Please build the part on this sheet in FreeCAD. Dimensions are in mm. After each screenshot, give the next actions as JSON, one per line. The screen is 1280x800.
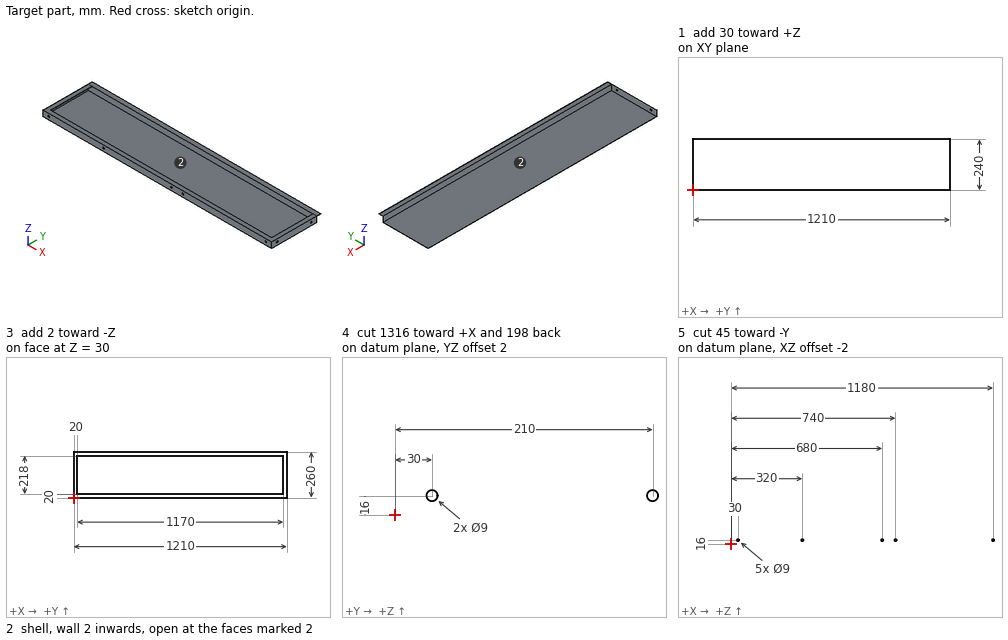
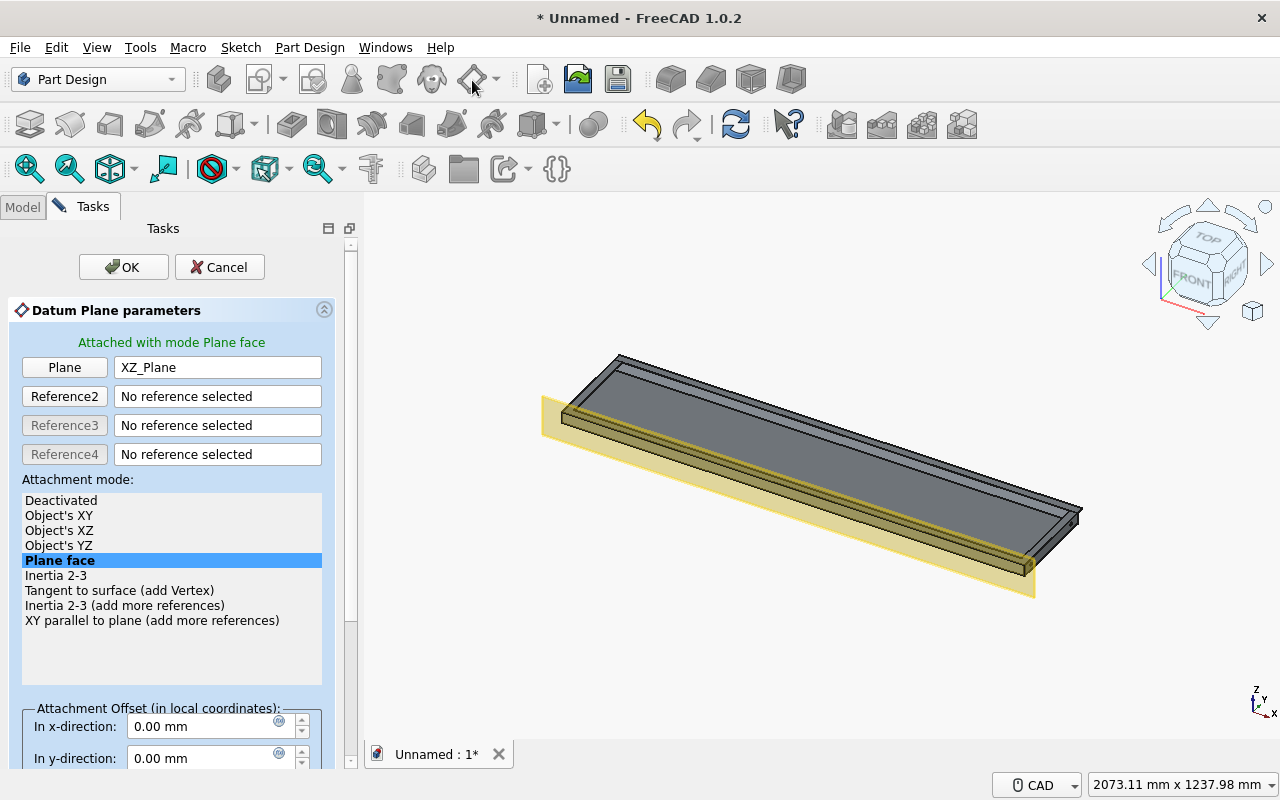
{"action": "scroll", "coordinate": [351, 503], "scroll_direction": "down", "scroll_amount": 2}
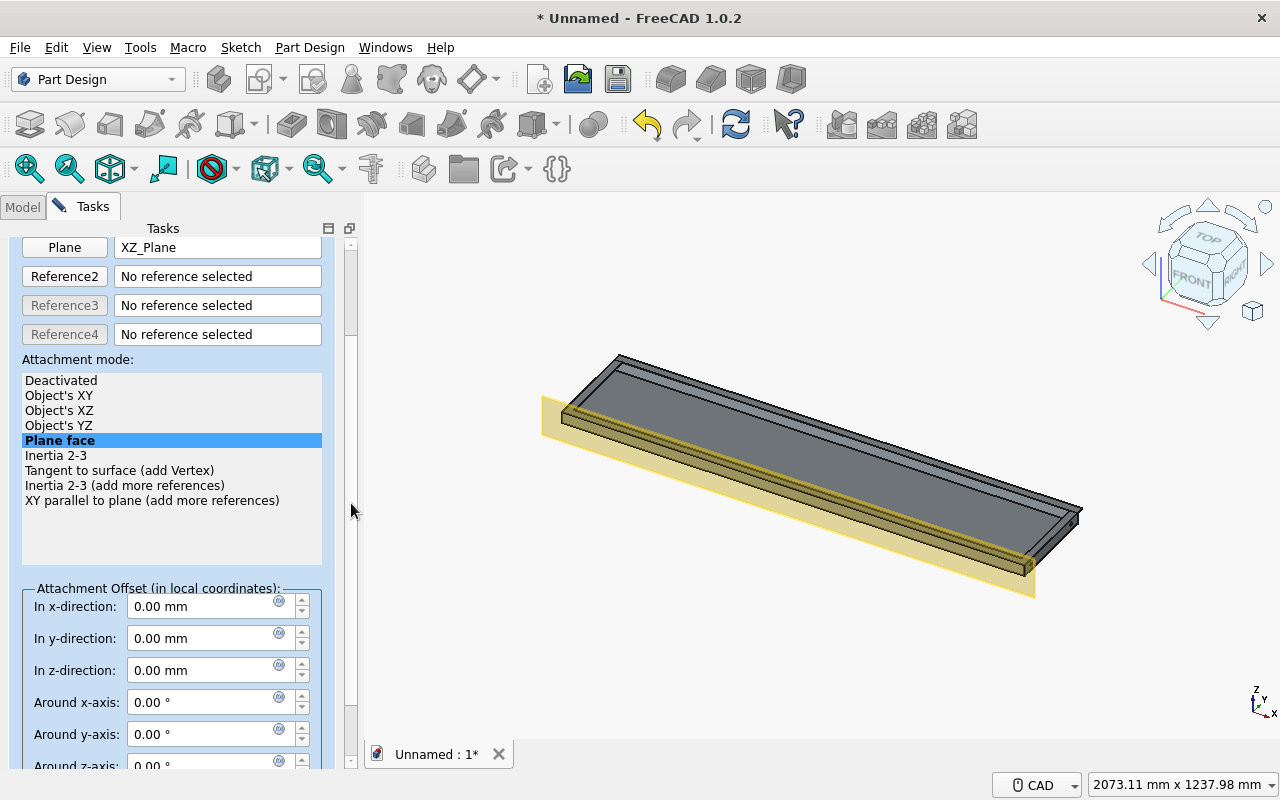
{"action": "triple_click", "coordinate": [210, 670]}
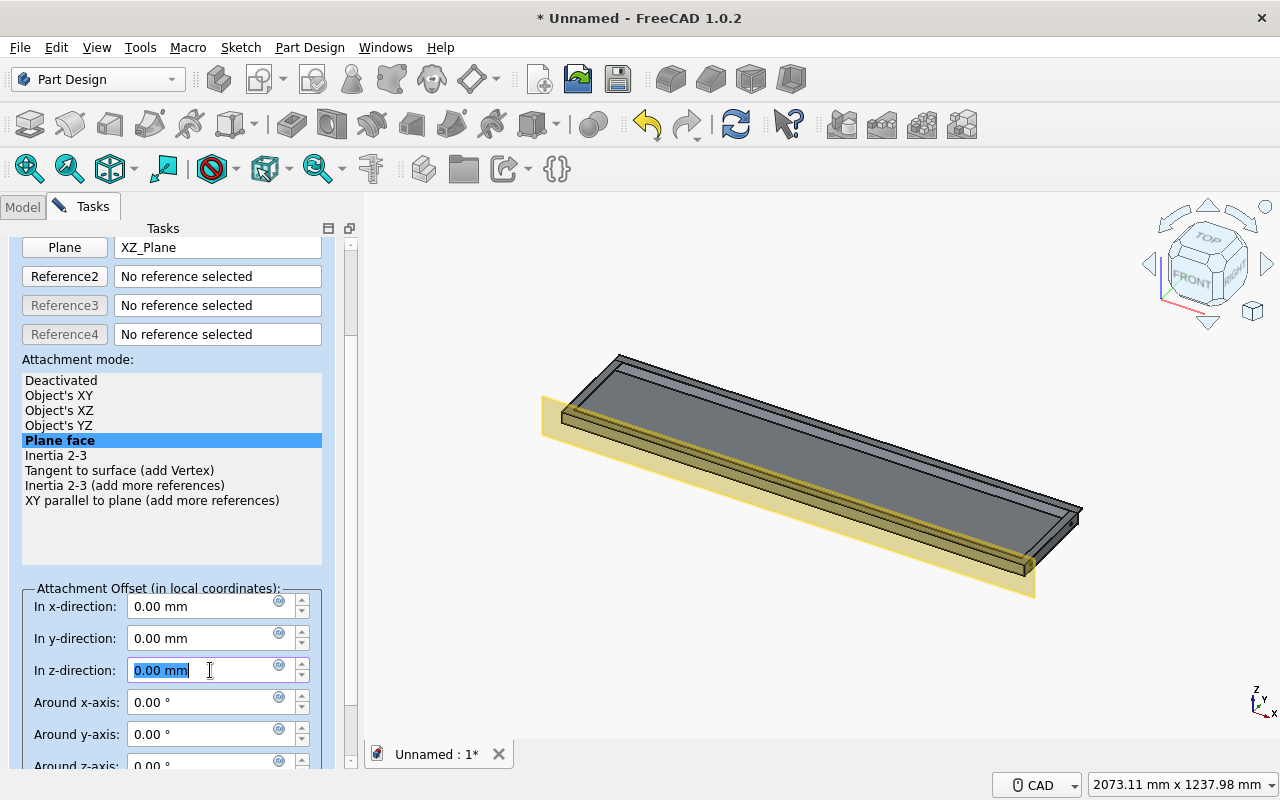
{"action": "type", "text": "-2"}
{"action": "key", "text": "Tab"}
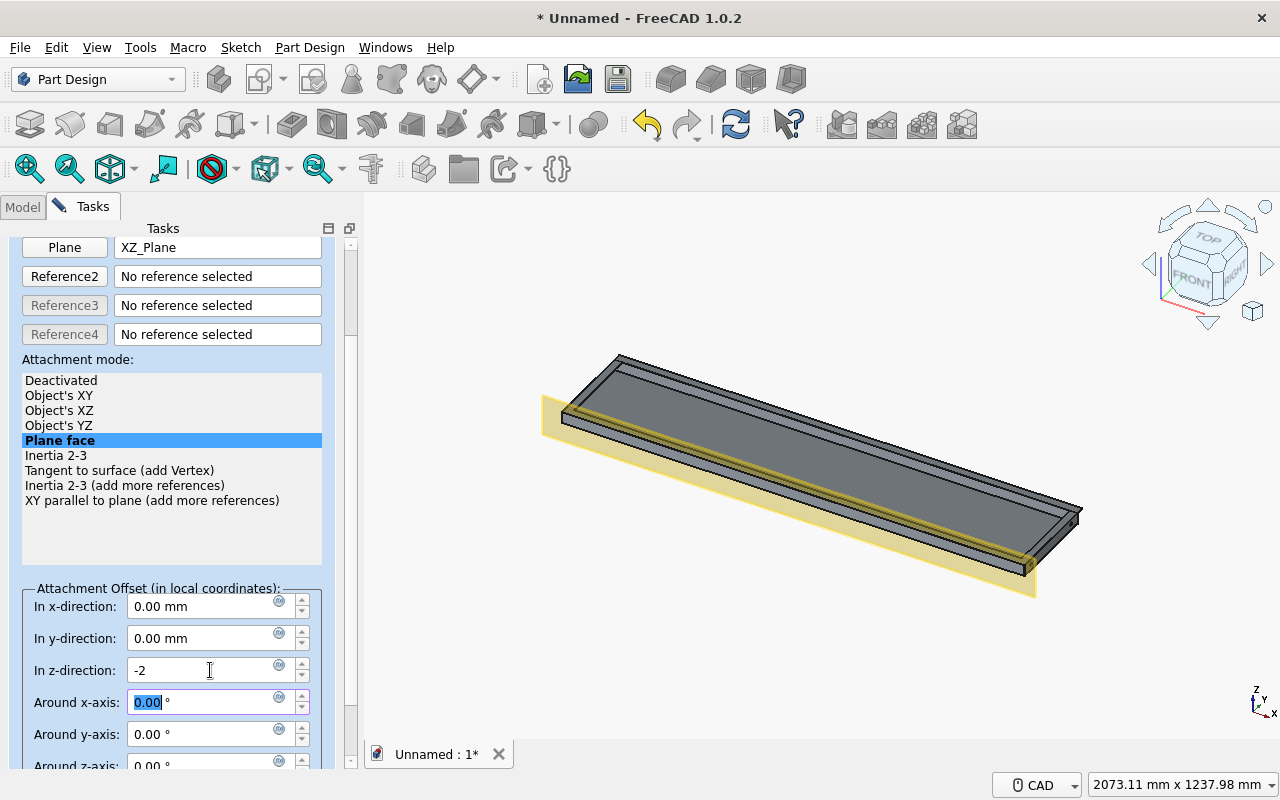
{"action": "scroll", "coordinate": [351, 503], "scroll_direction": "up", "scroll_amount": 3}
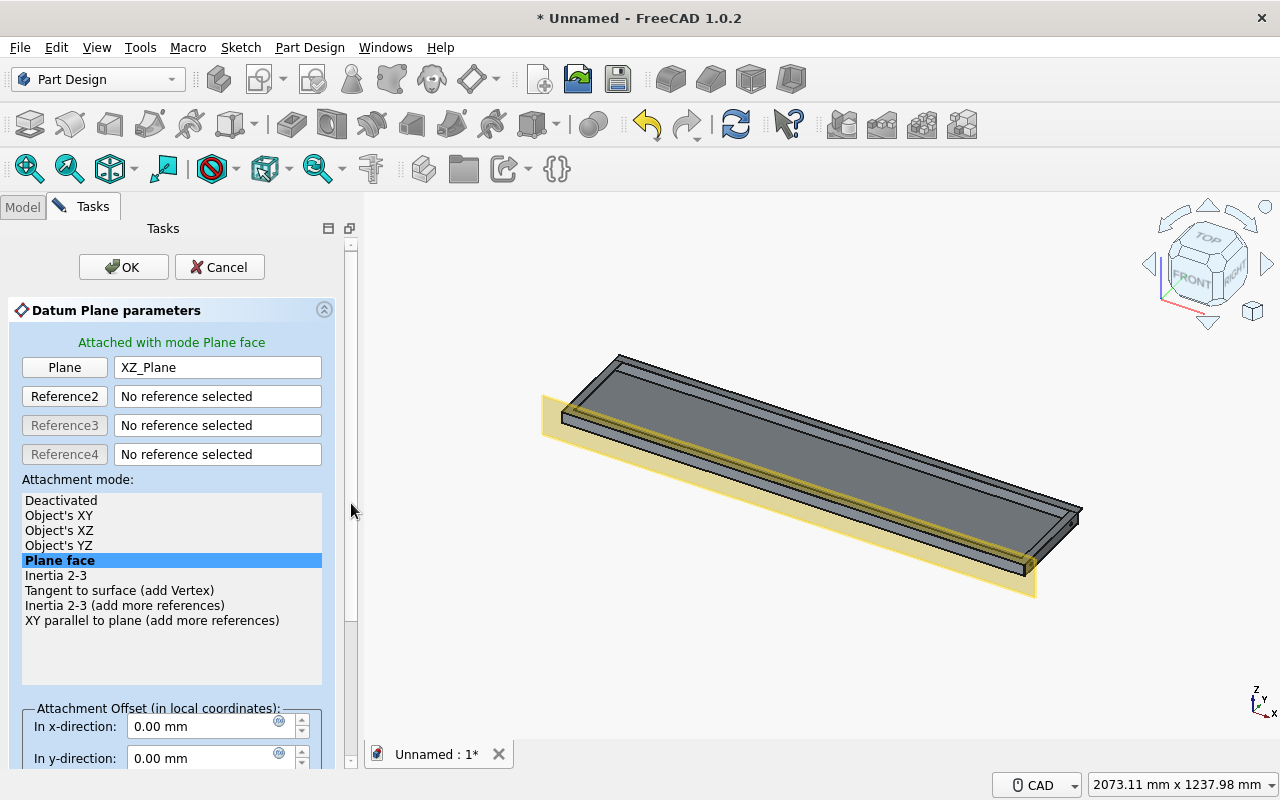
{"action": "left_click", "coordinate": [124, 267]}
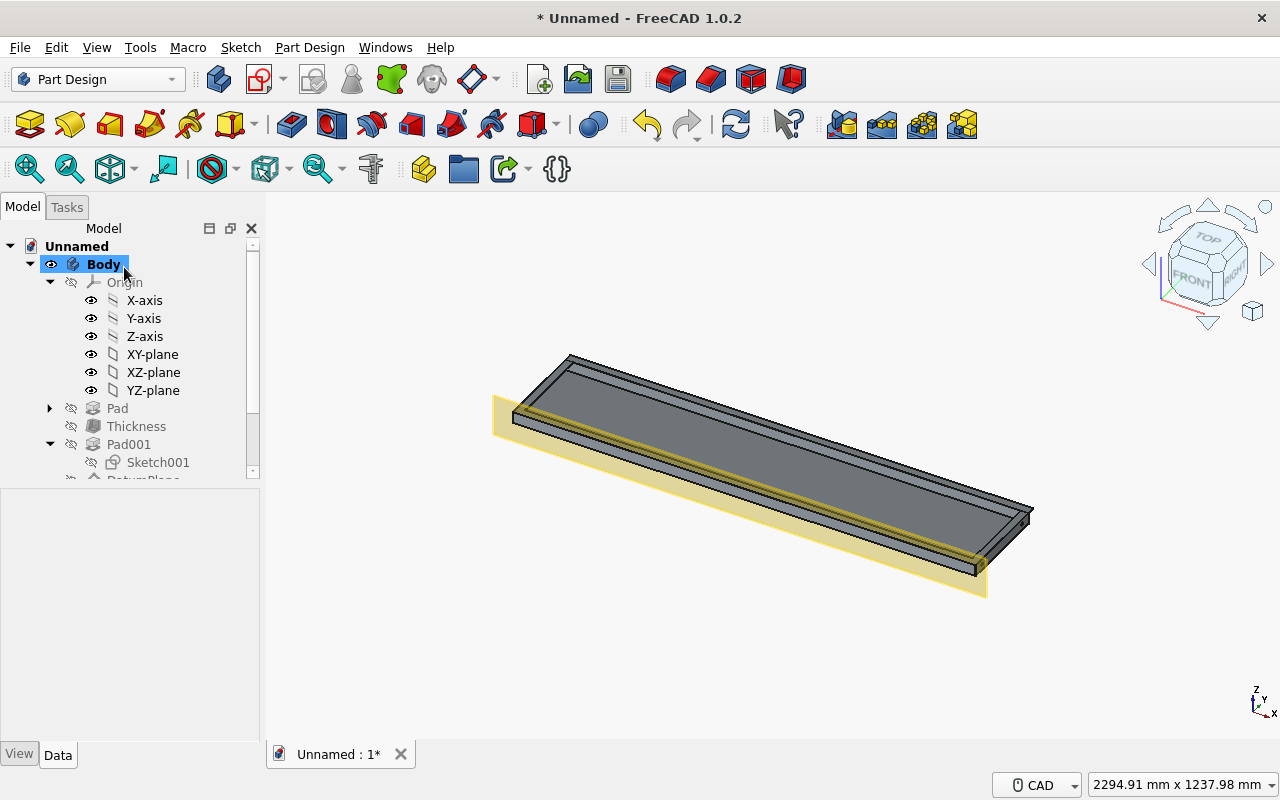
{"action": "scroll", "coordinate": [100, 350], "scroll_direction": "down", "scroll_amount": 3}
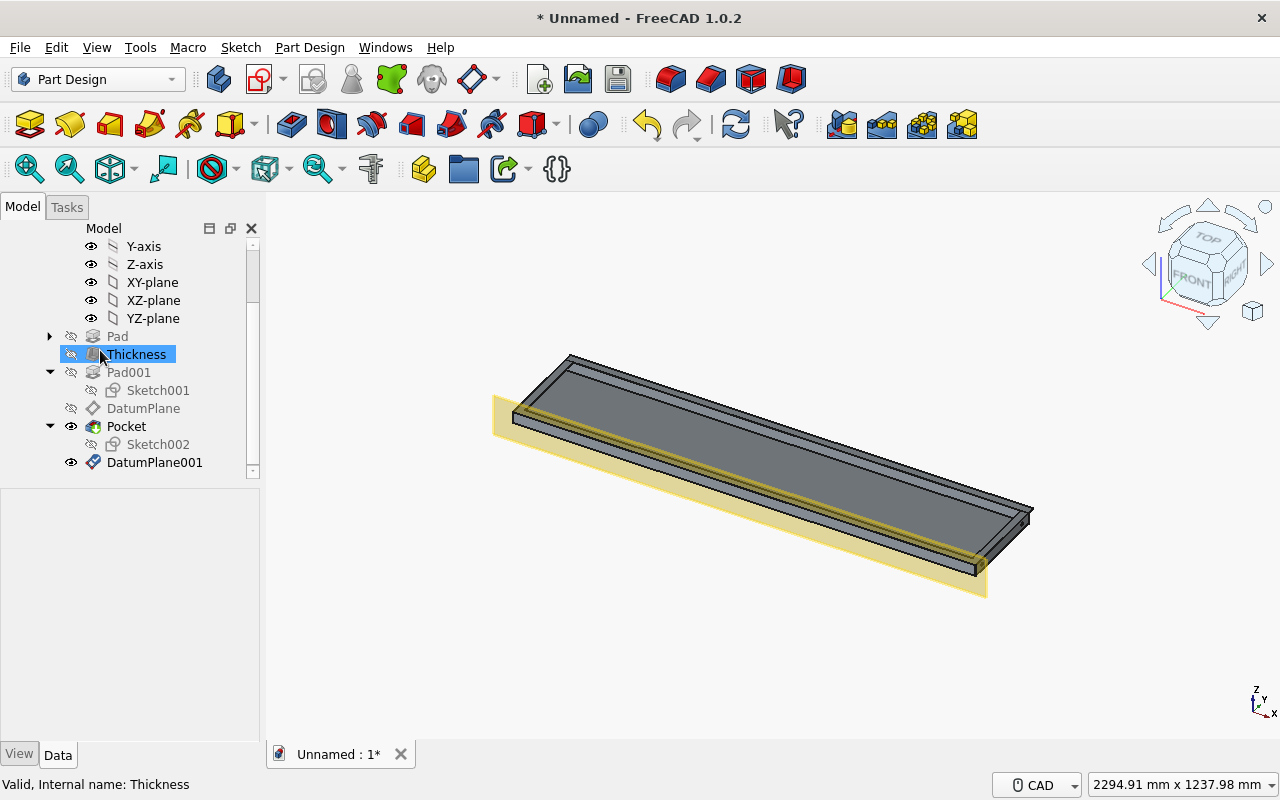
{"action": "left_click", "coordinate": [116, 462]}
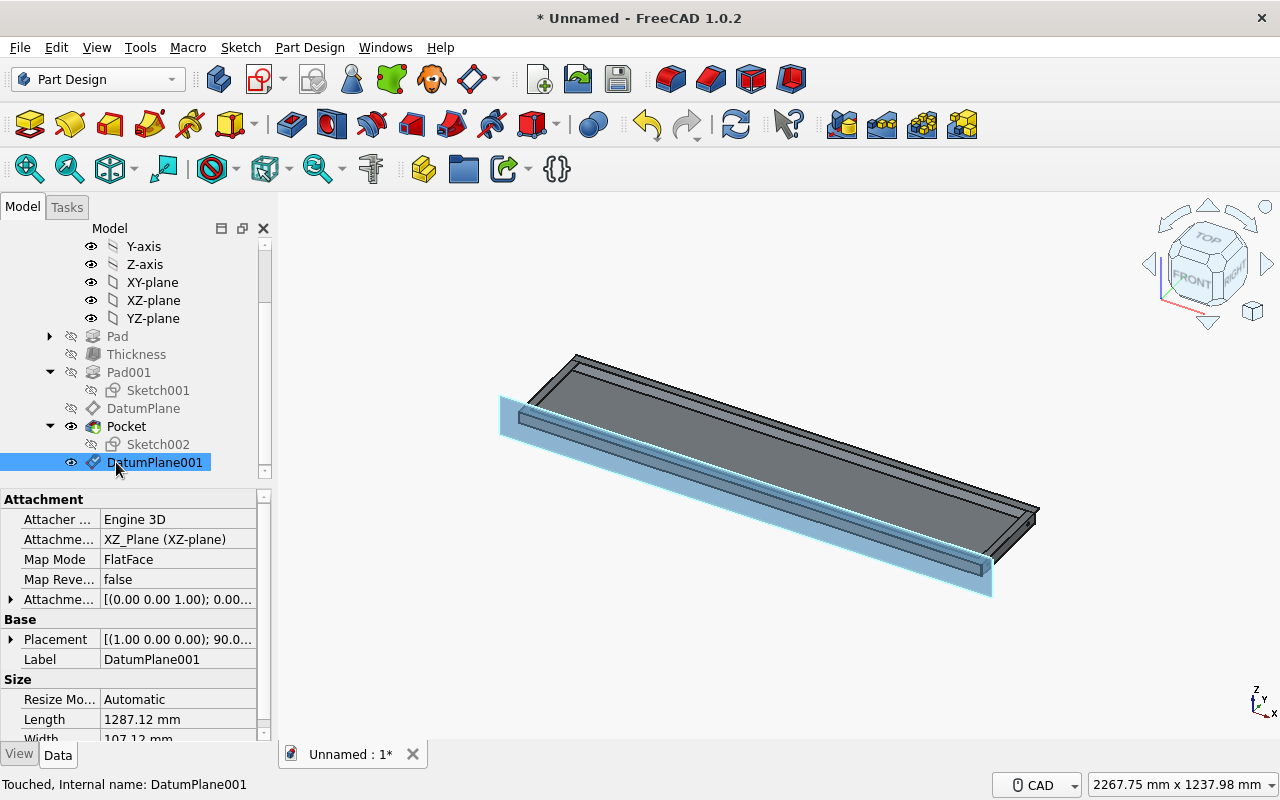
{"action": "left_click", "coordinate": [260, 80]}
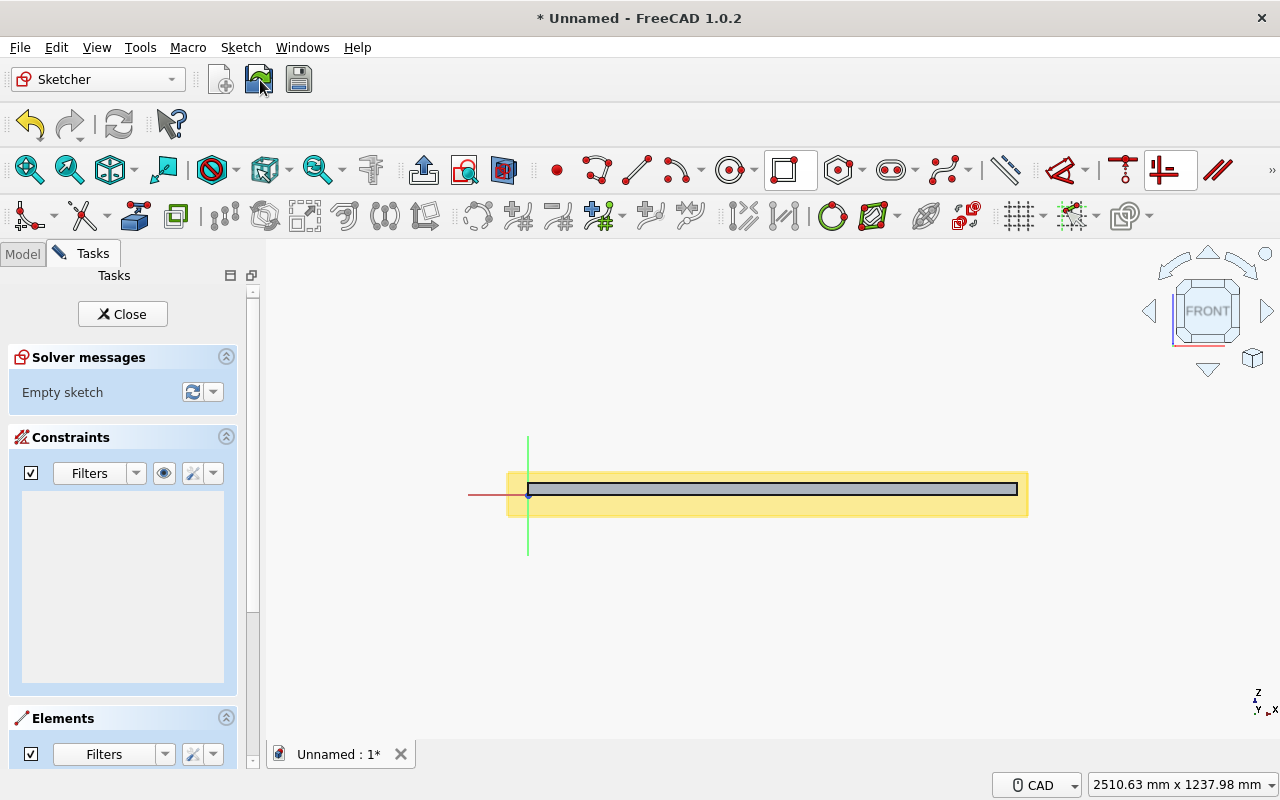
{"action": "left_click", "coordinate": [504, 170]}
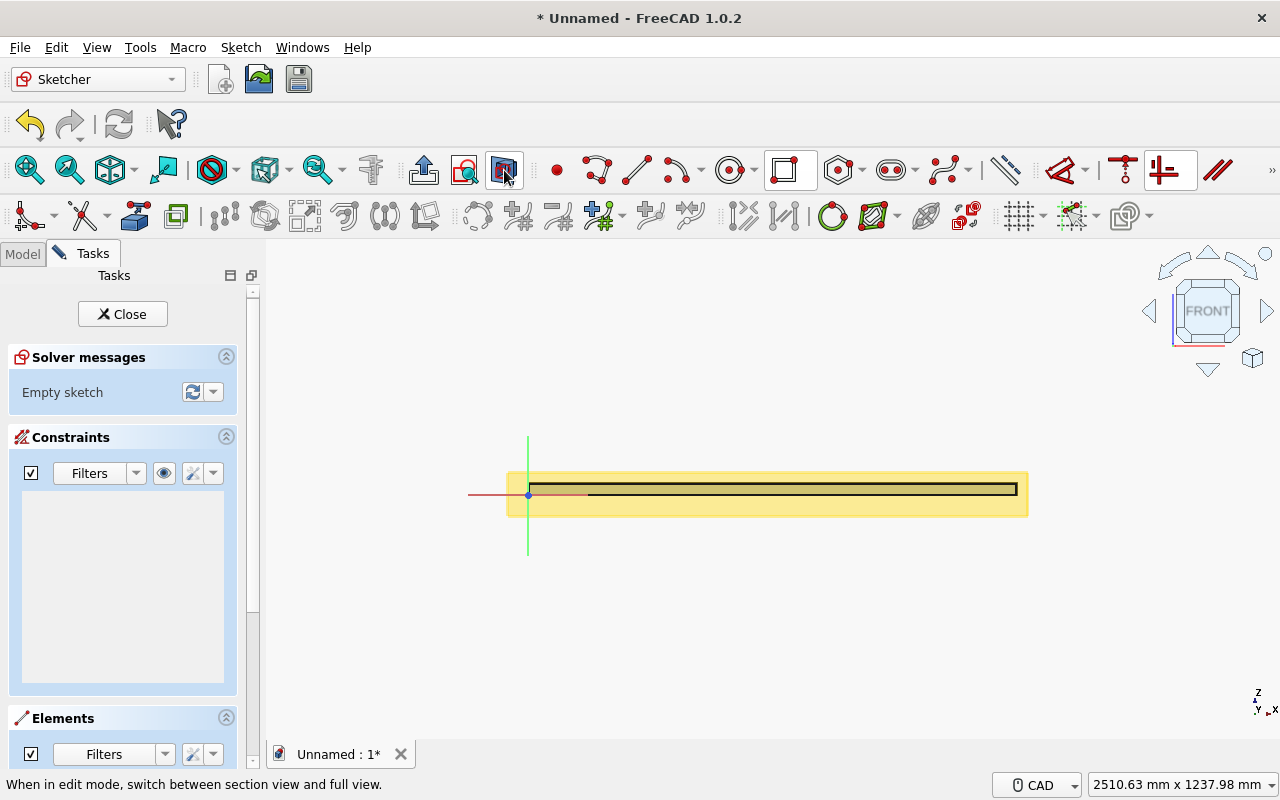
{"action": "left_click", "coordinate": [730, 170]}